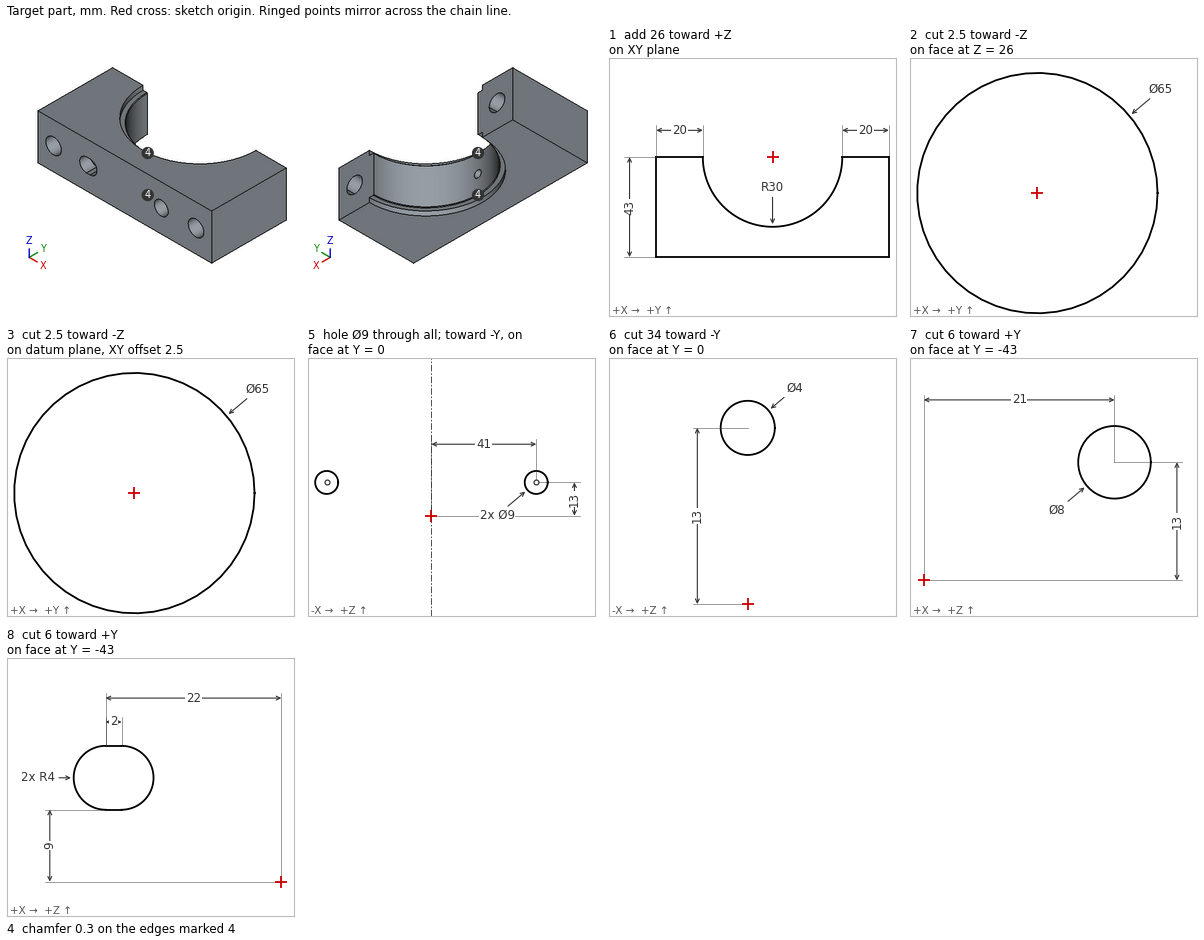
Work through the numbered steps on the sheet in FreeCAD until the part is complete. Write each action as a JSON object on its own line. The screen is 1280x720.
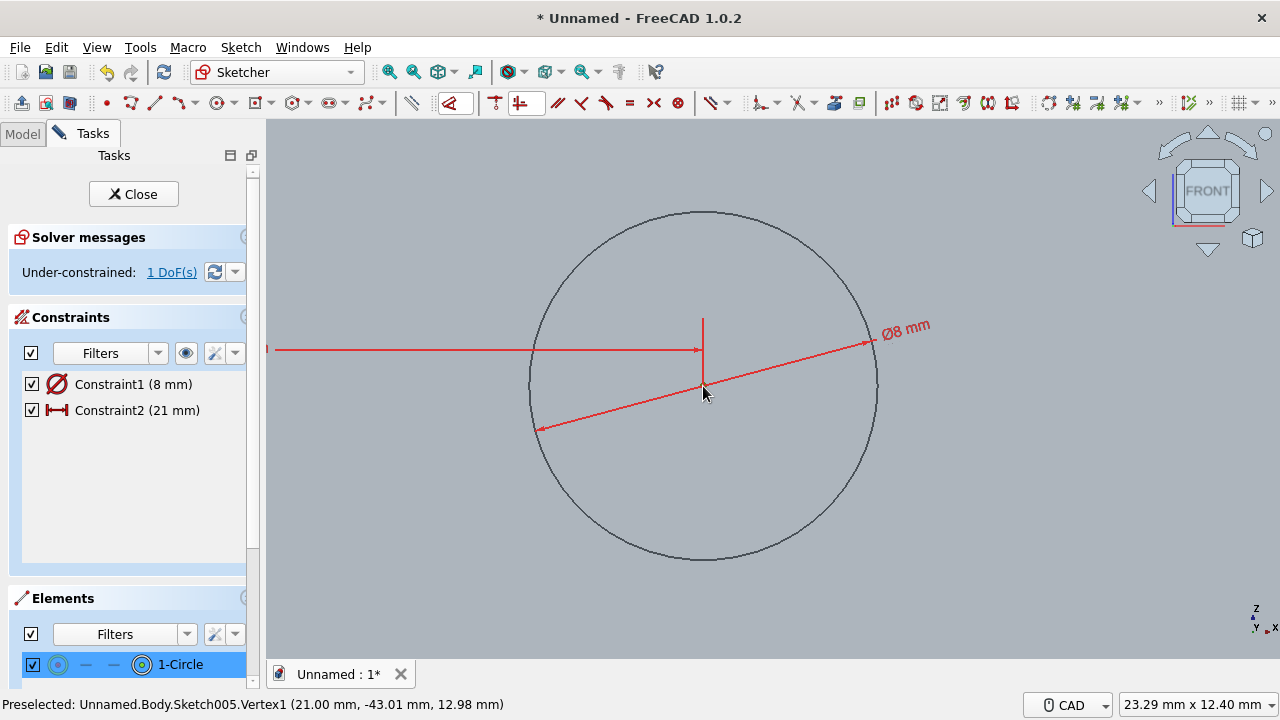
{"action": "key", "text": "i"}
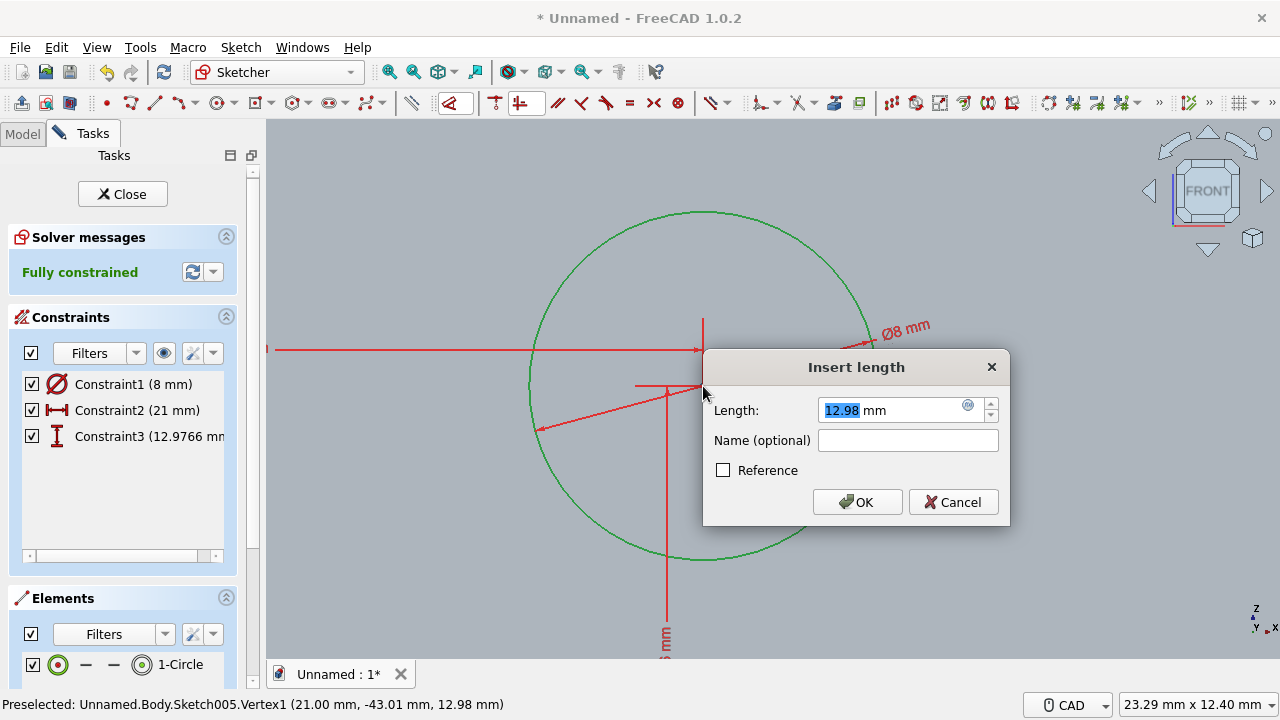
{"action": "type", "text": "13"}
{"action": "key", "text": "Return"}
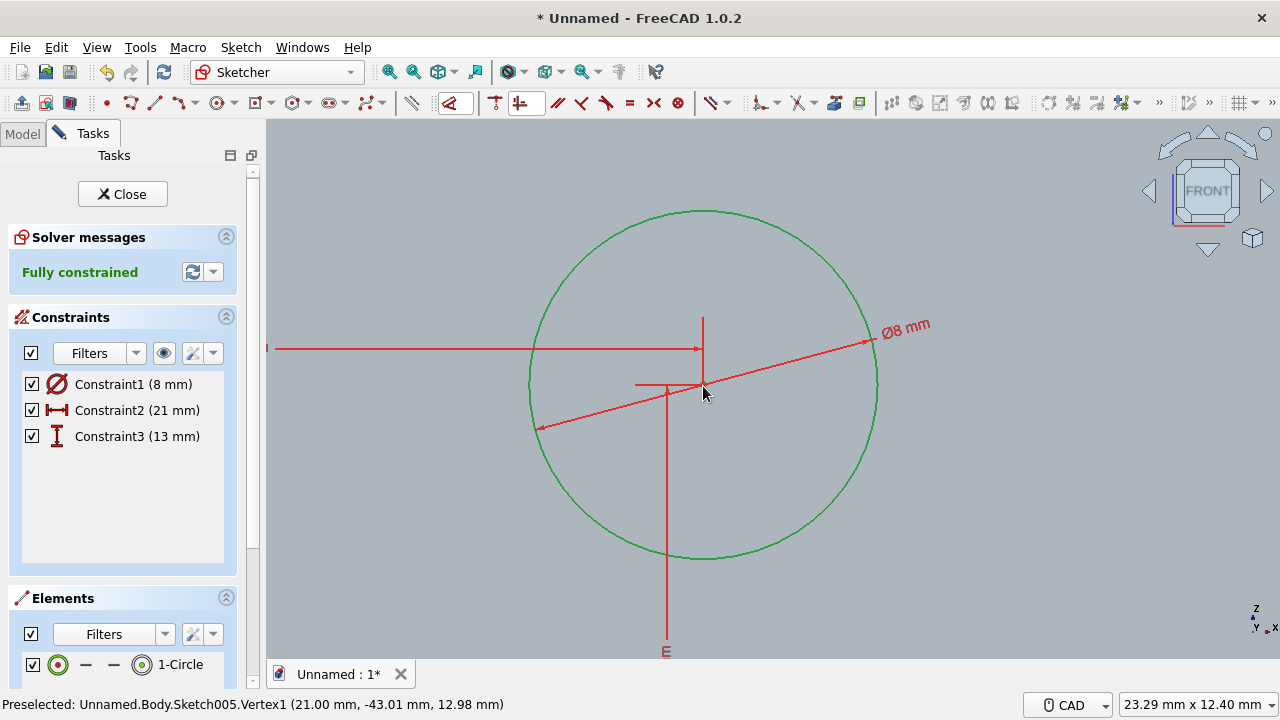
{"action": "left_click", "coordinate": [123, 194]}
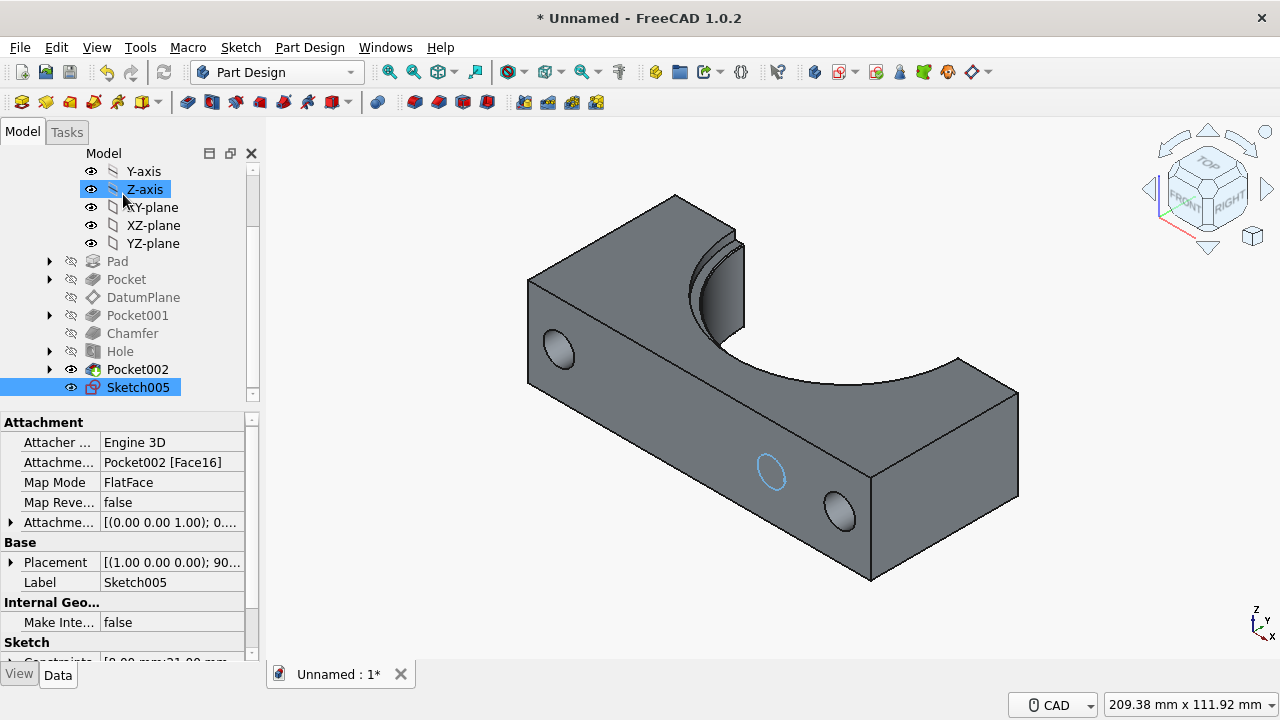
{"action": "left_click", "coordinate": [188, 102]}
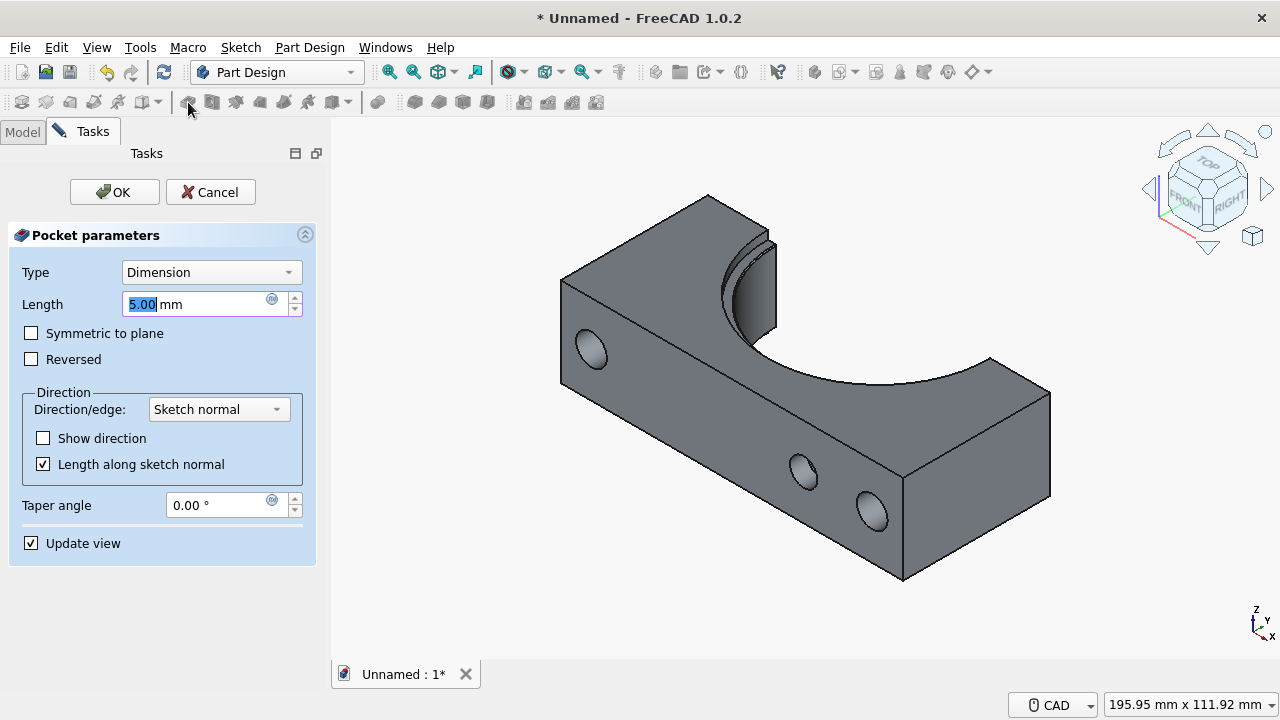
{"action": "type", "text": "6"}
{"action": "key", "text": "Tab"}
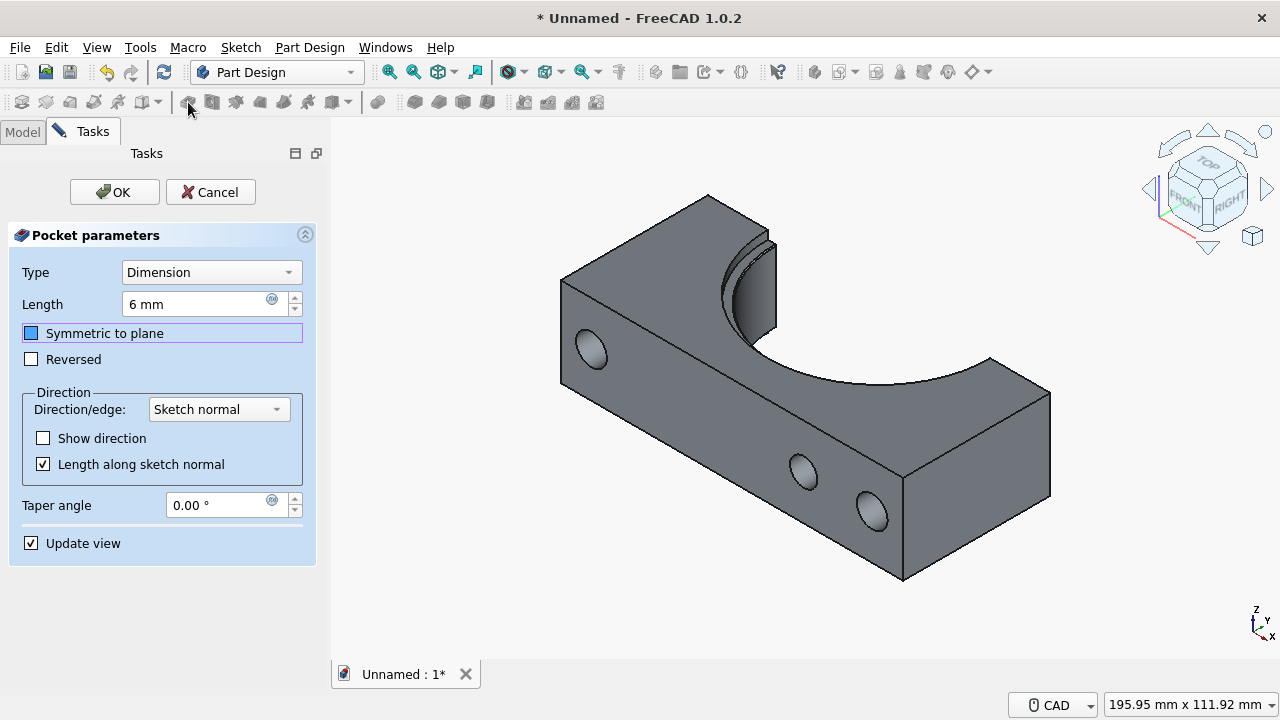
{"action": "left_click", "coordinate": [115, 192]}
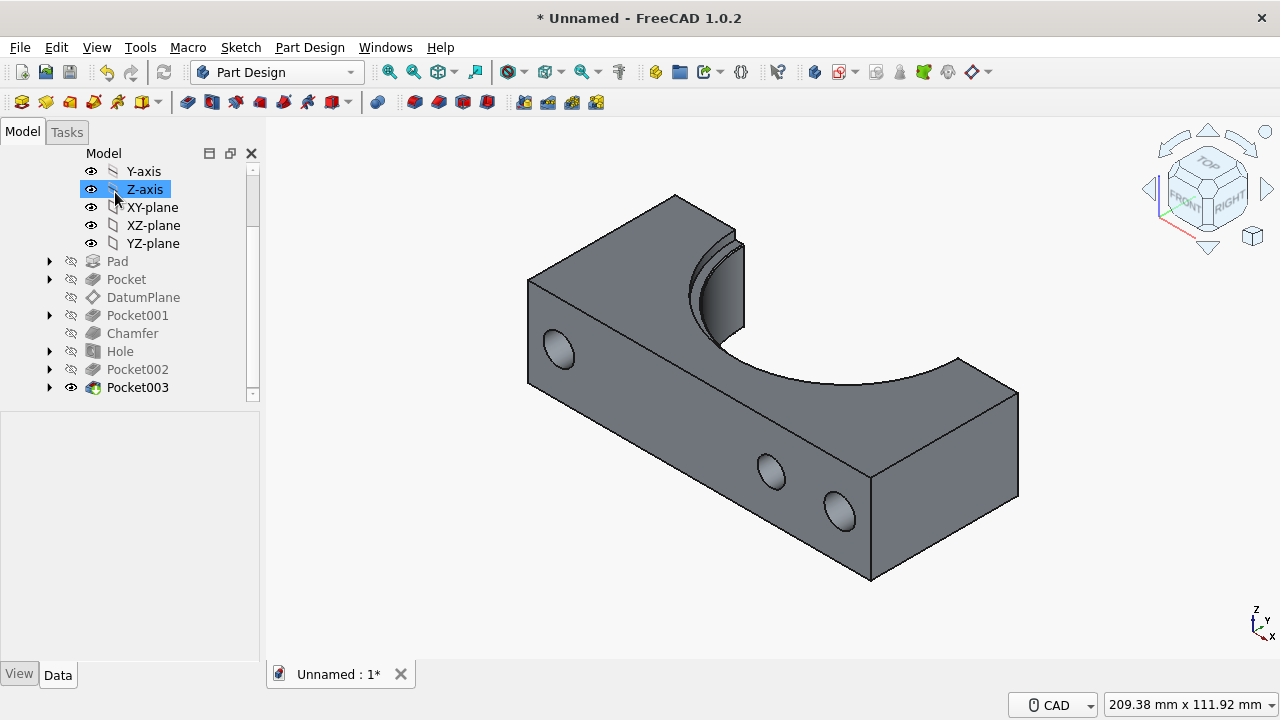
{"action": "left_click", "coordinate": [699, 430]}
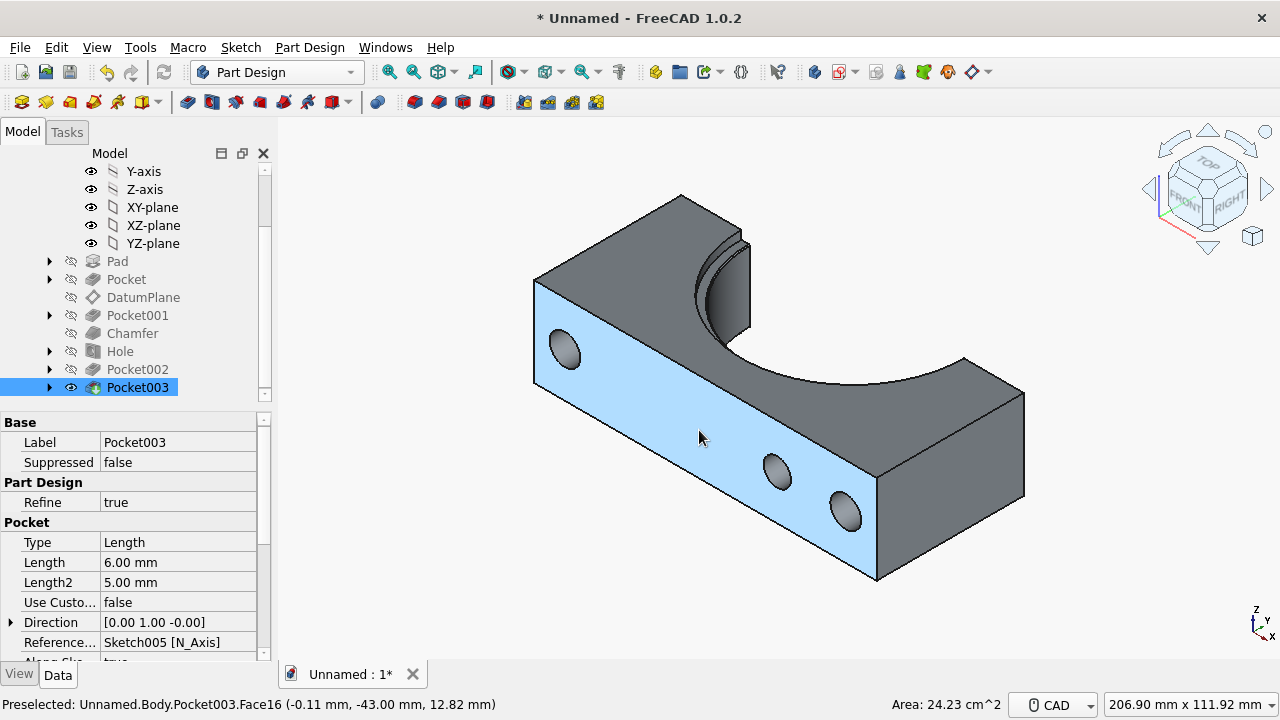
{"action": "left_click", "coordinate": [840, 72]}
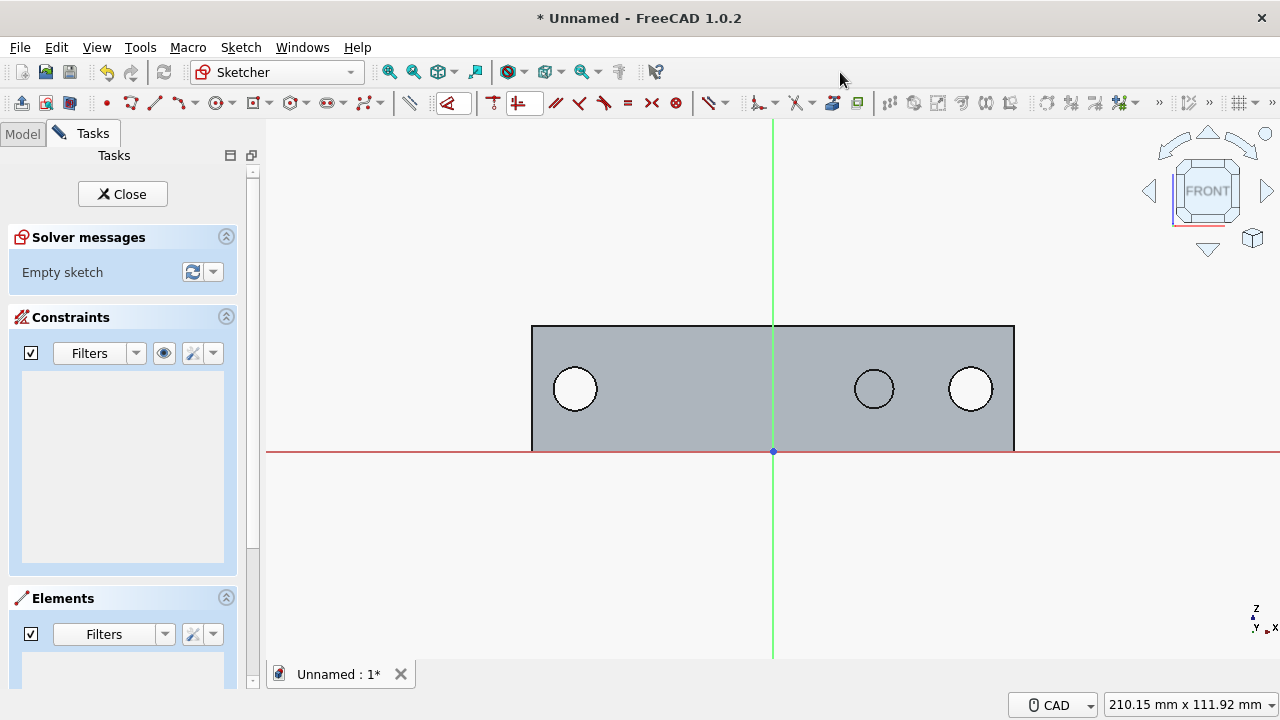
{"action": "scroll", "coordinate": [668, 389], "scroll_direction": "up", "scroll_amount": 11}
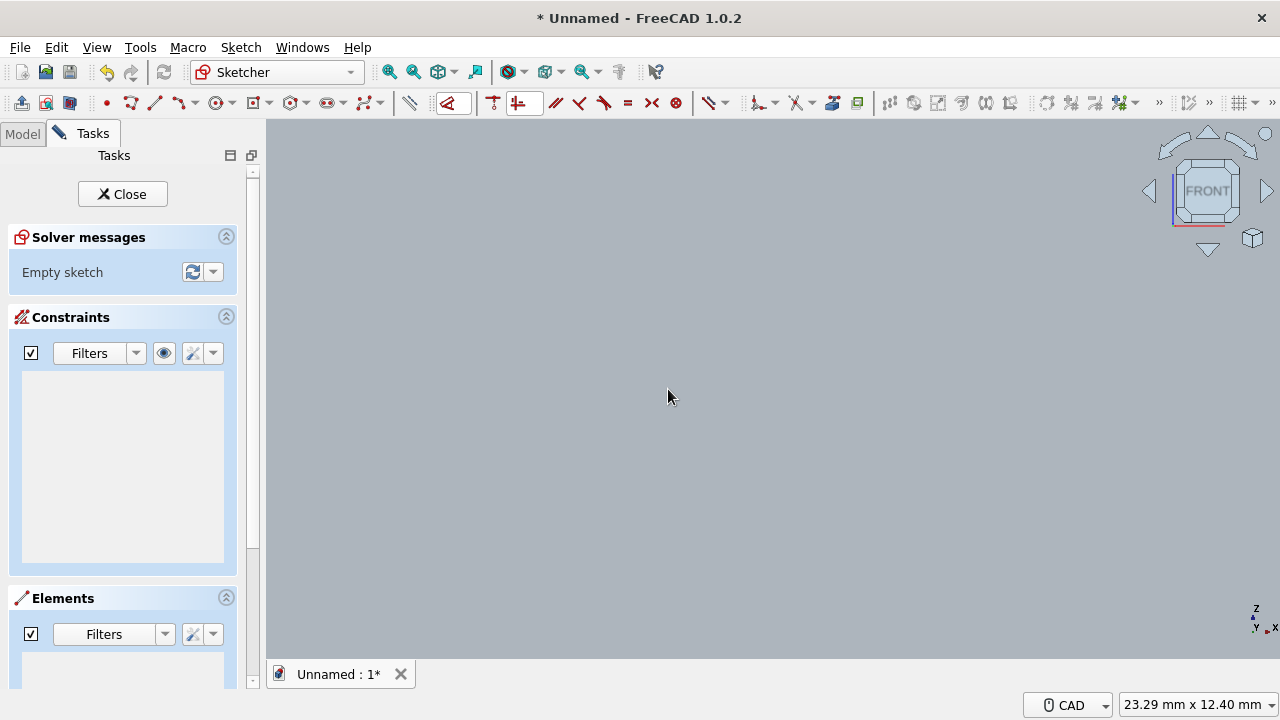
{"action": "left_click", "coordinate": [328, 104]}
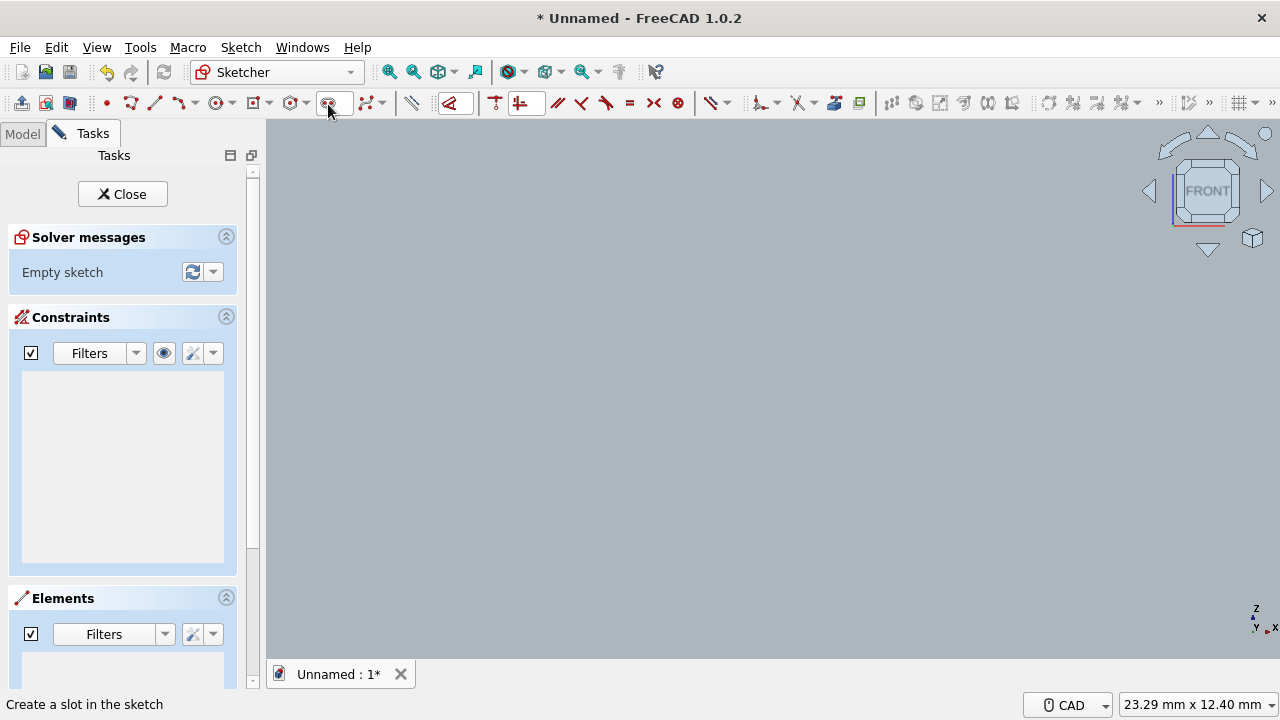
{"action": "left_click", "coordinate": [654, 385]}